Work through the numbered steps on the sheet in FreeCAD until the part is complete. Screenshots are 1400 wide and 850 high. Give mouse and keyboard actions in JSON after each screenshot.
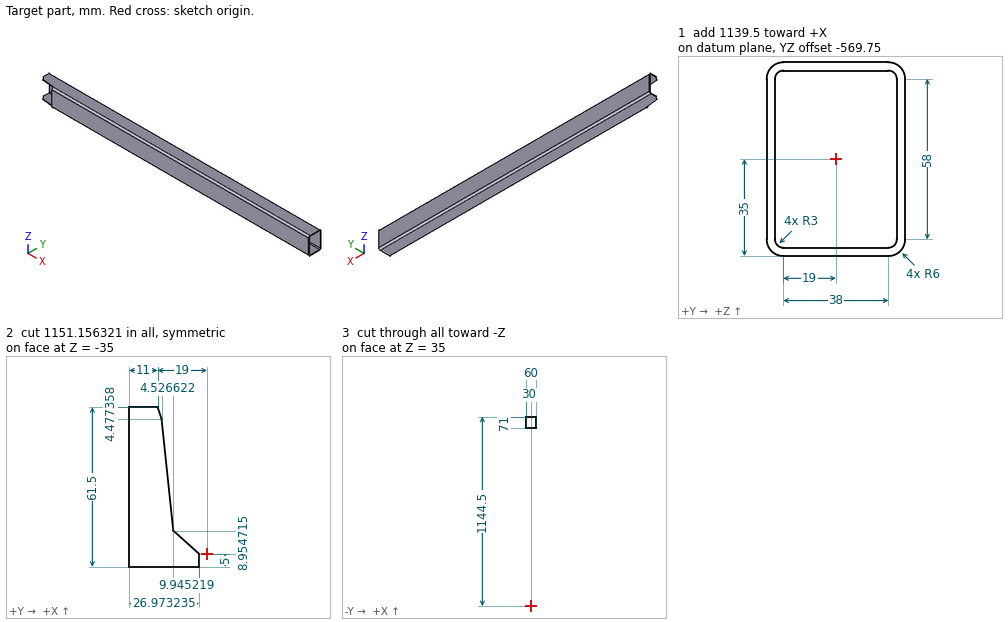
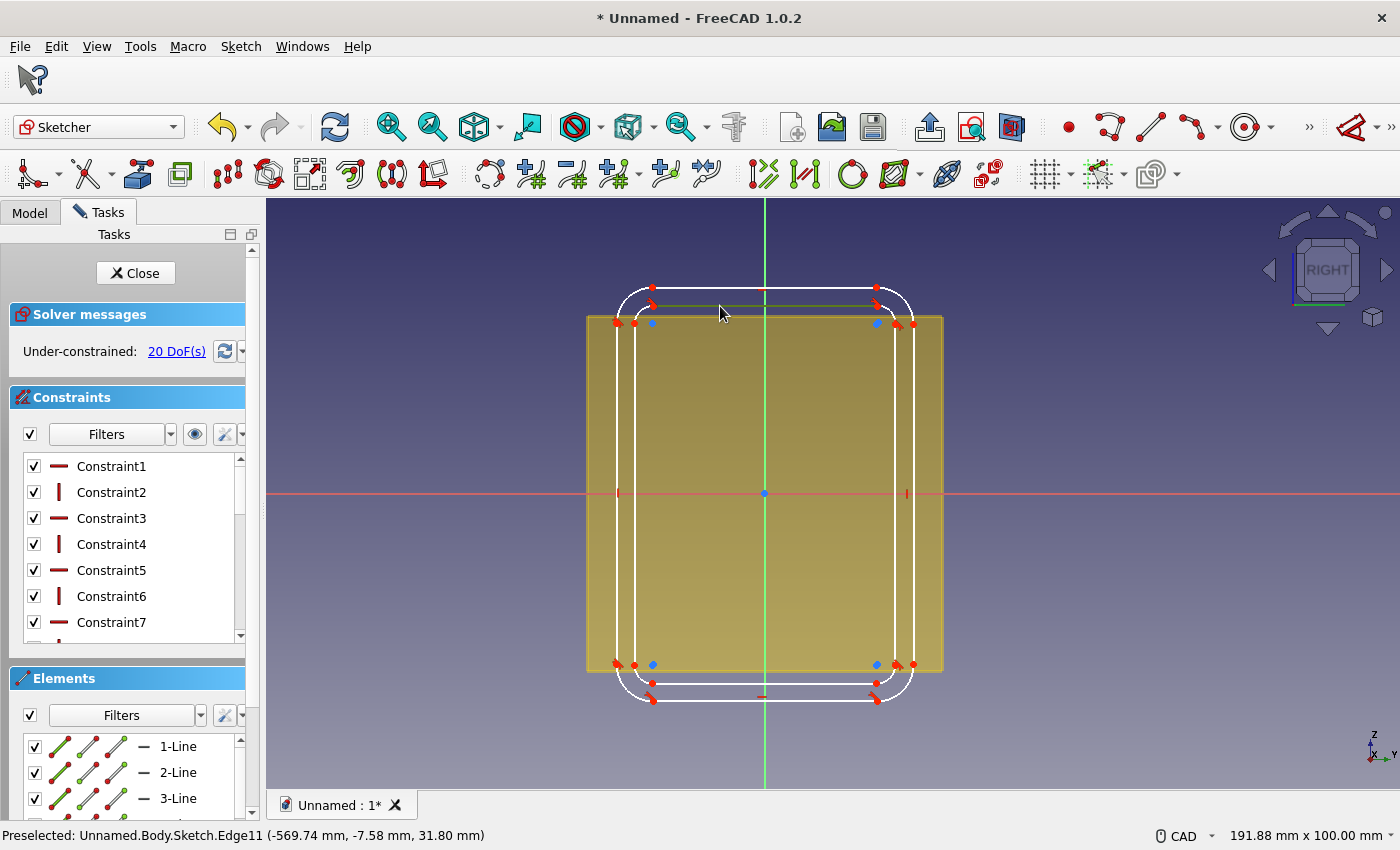
{"action": "left_click", "coordinate": [640, 311]}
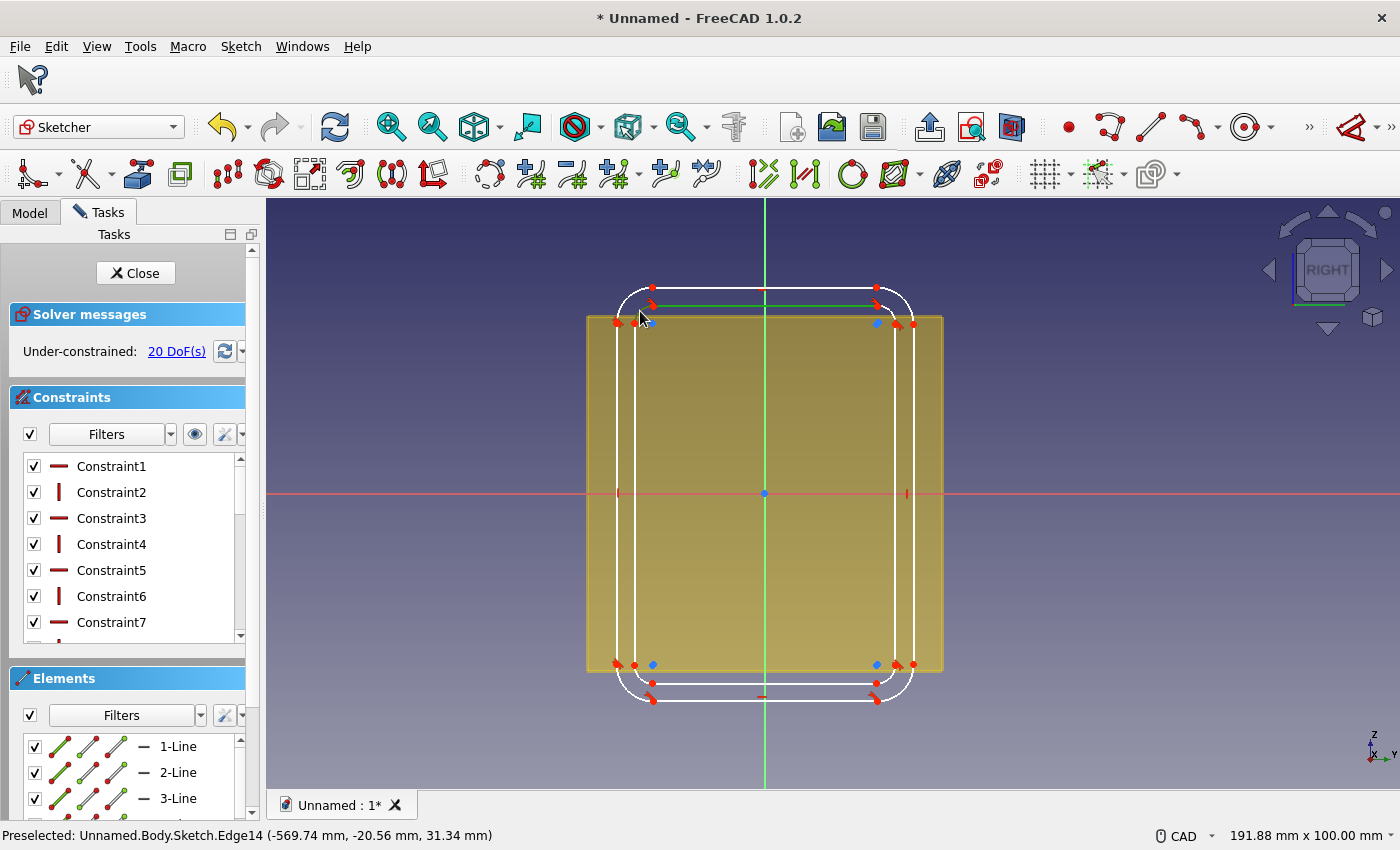
{"action": "key", "text": "t"}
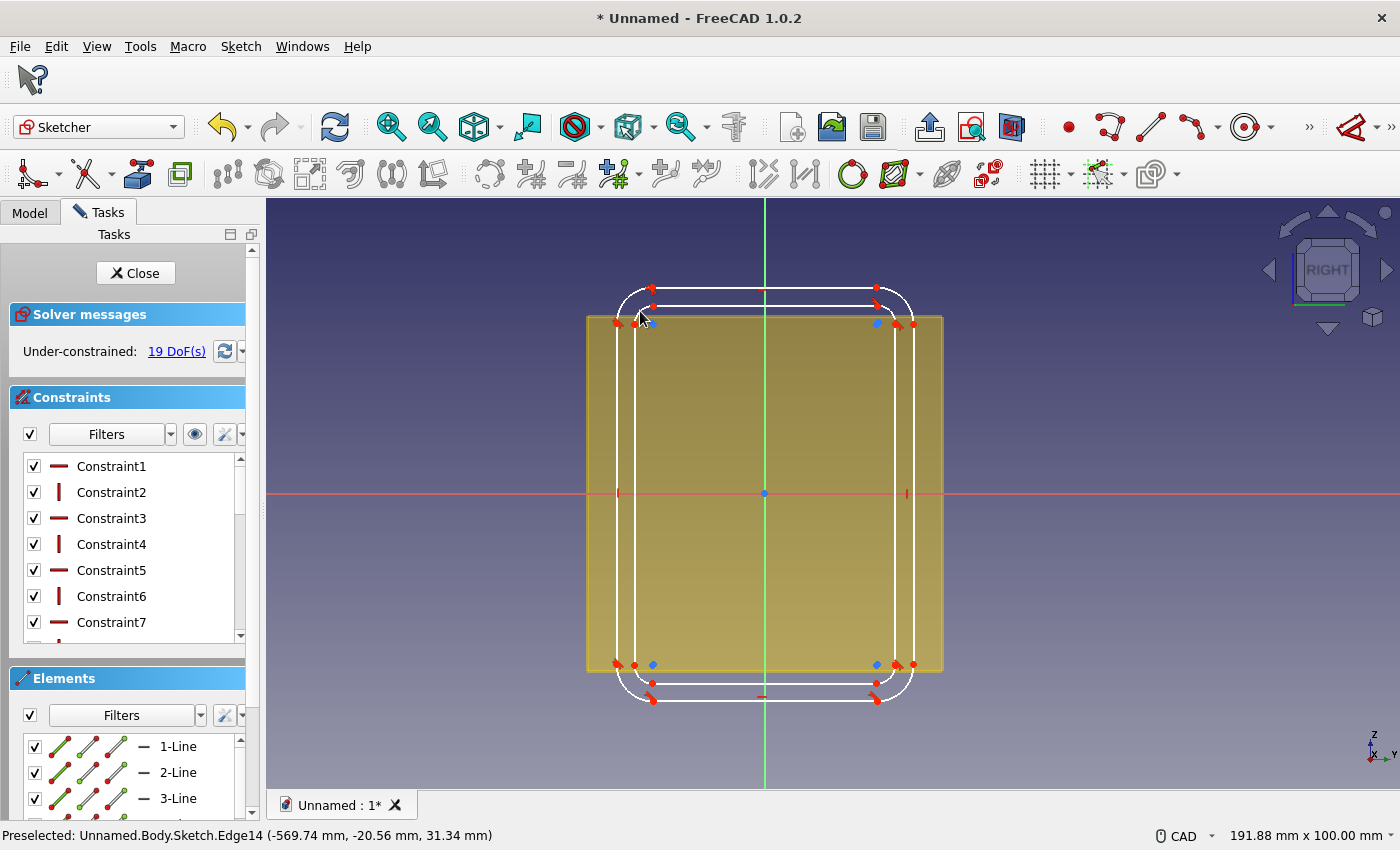
{"action": "left_click", "coordinate": [720, 306]}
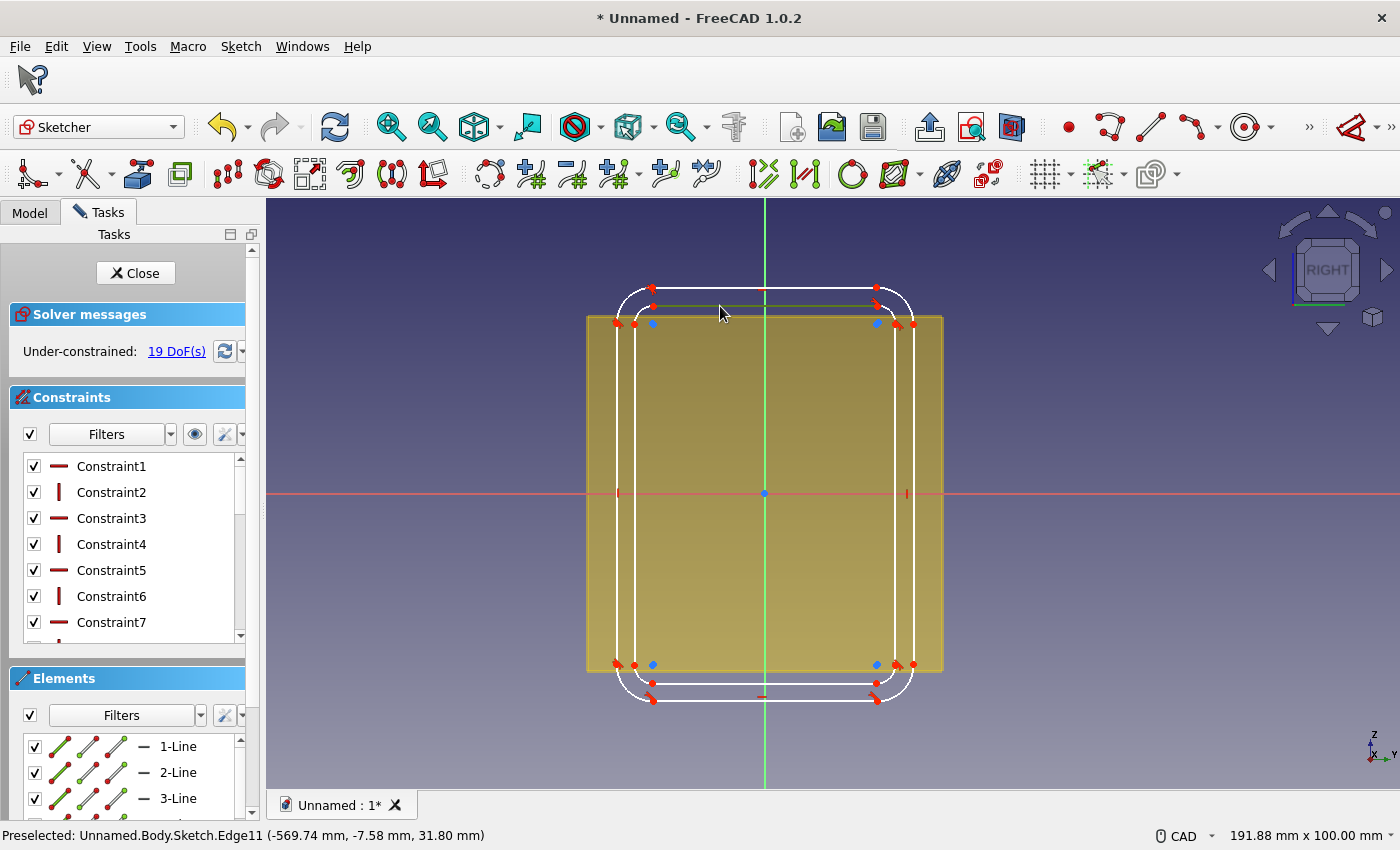
{"action": "left_click", "coordinate": [890, 311]}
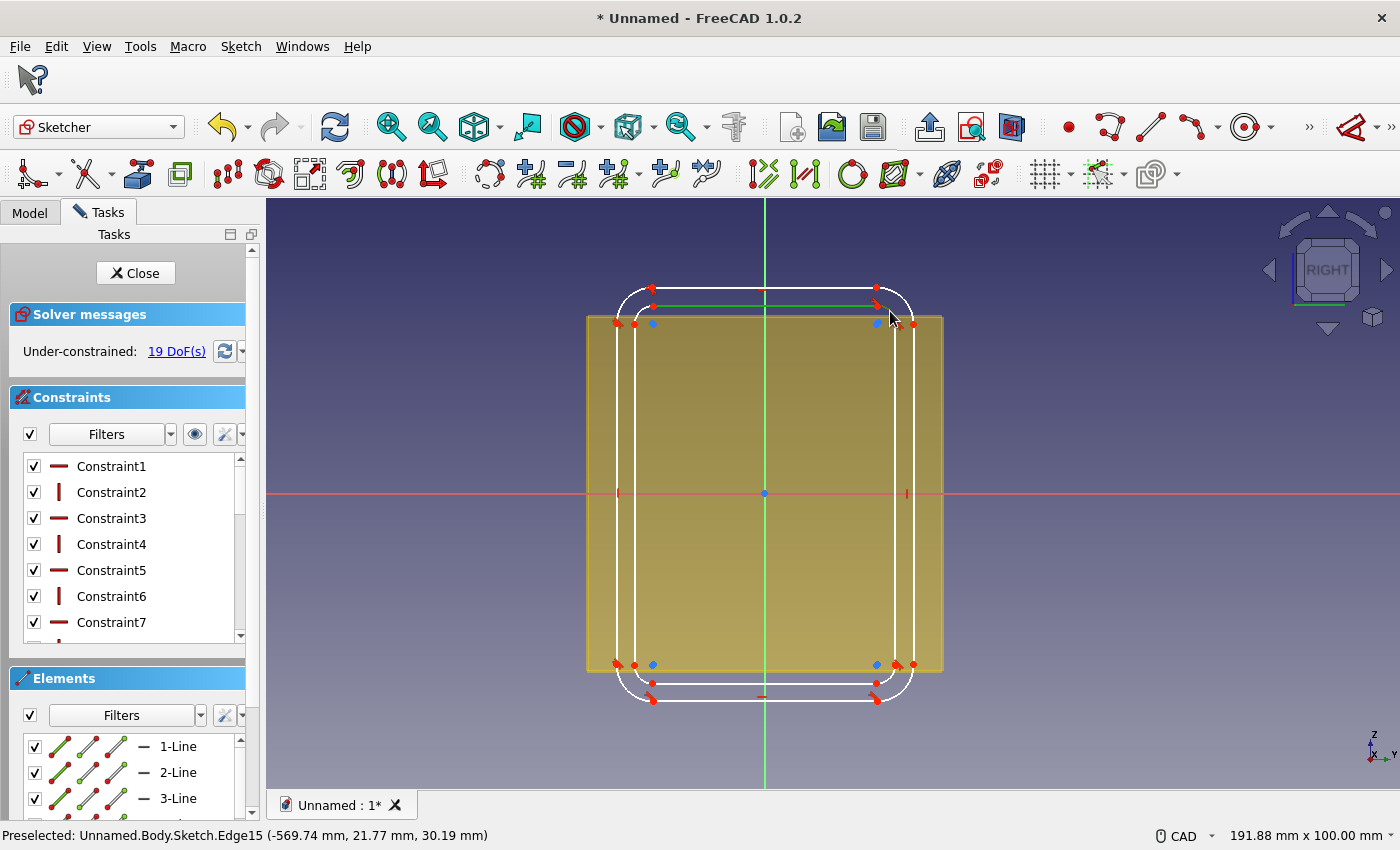
{"action": "key", "text": "t"}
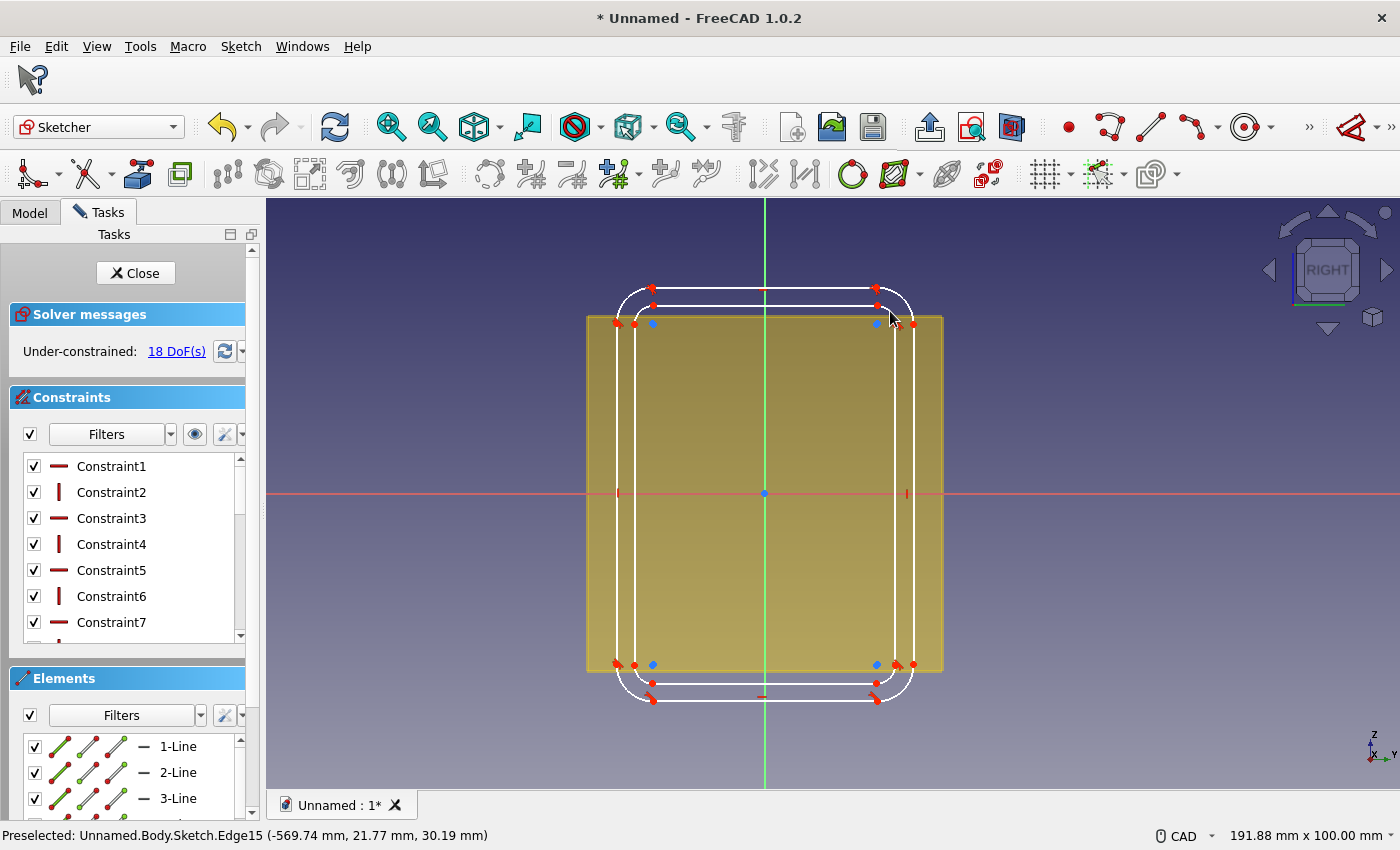
{"action": "left_click", "coordinate": [895, 427]}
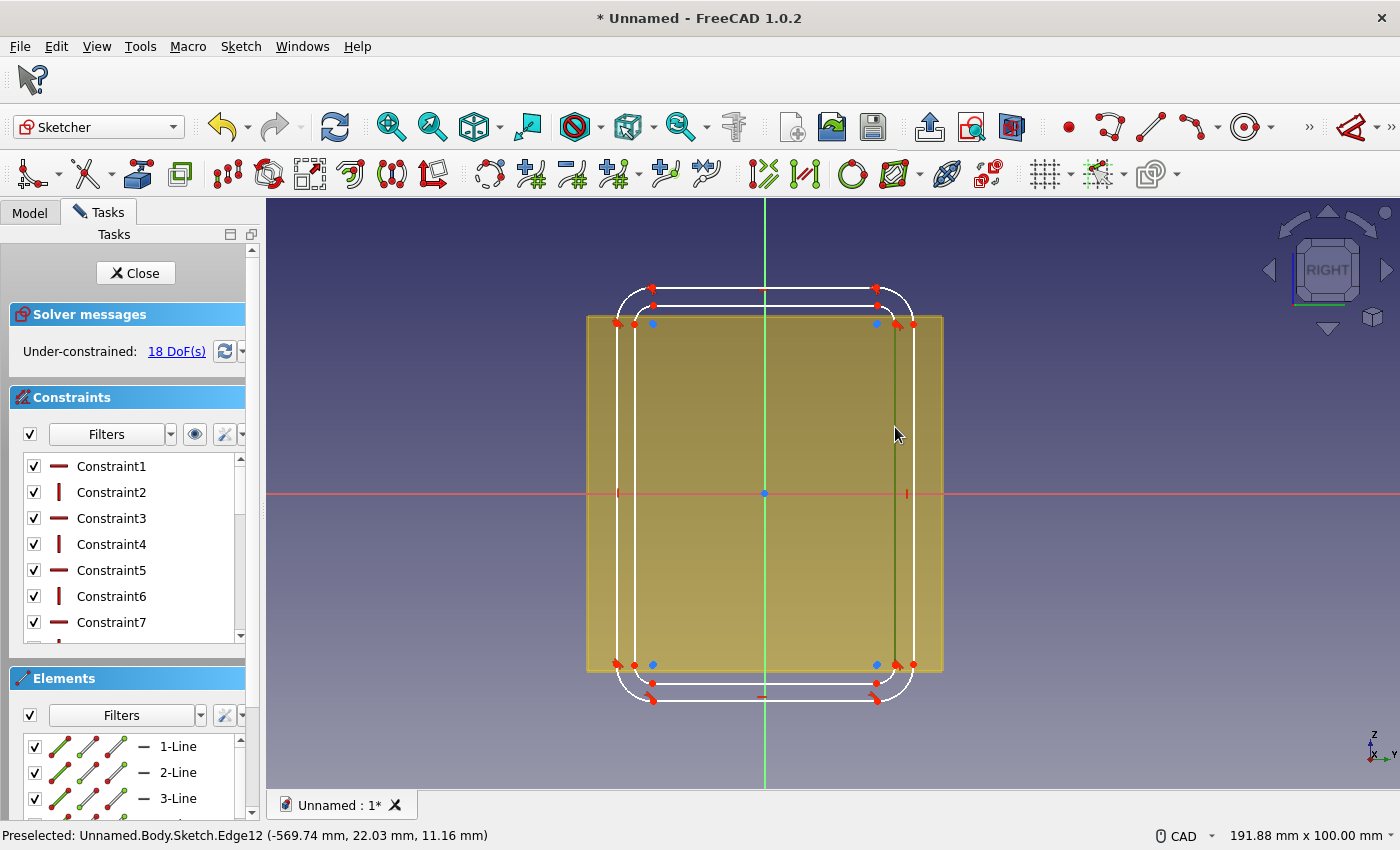
{"action": "left_click", "coordinate": [890, 311]}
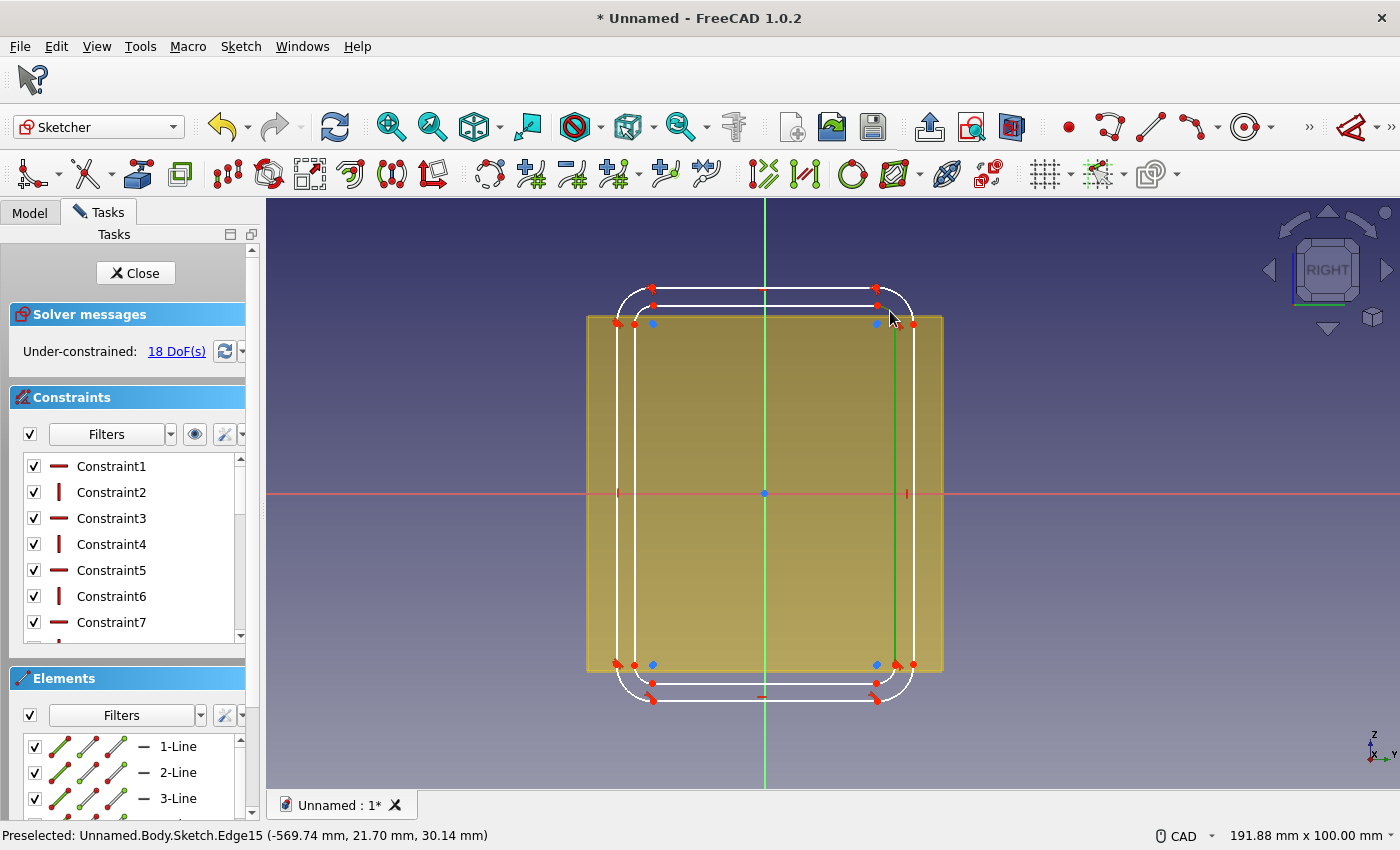
{"action": "key", "text": "t"}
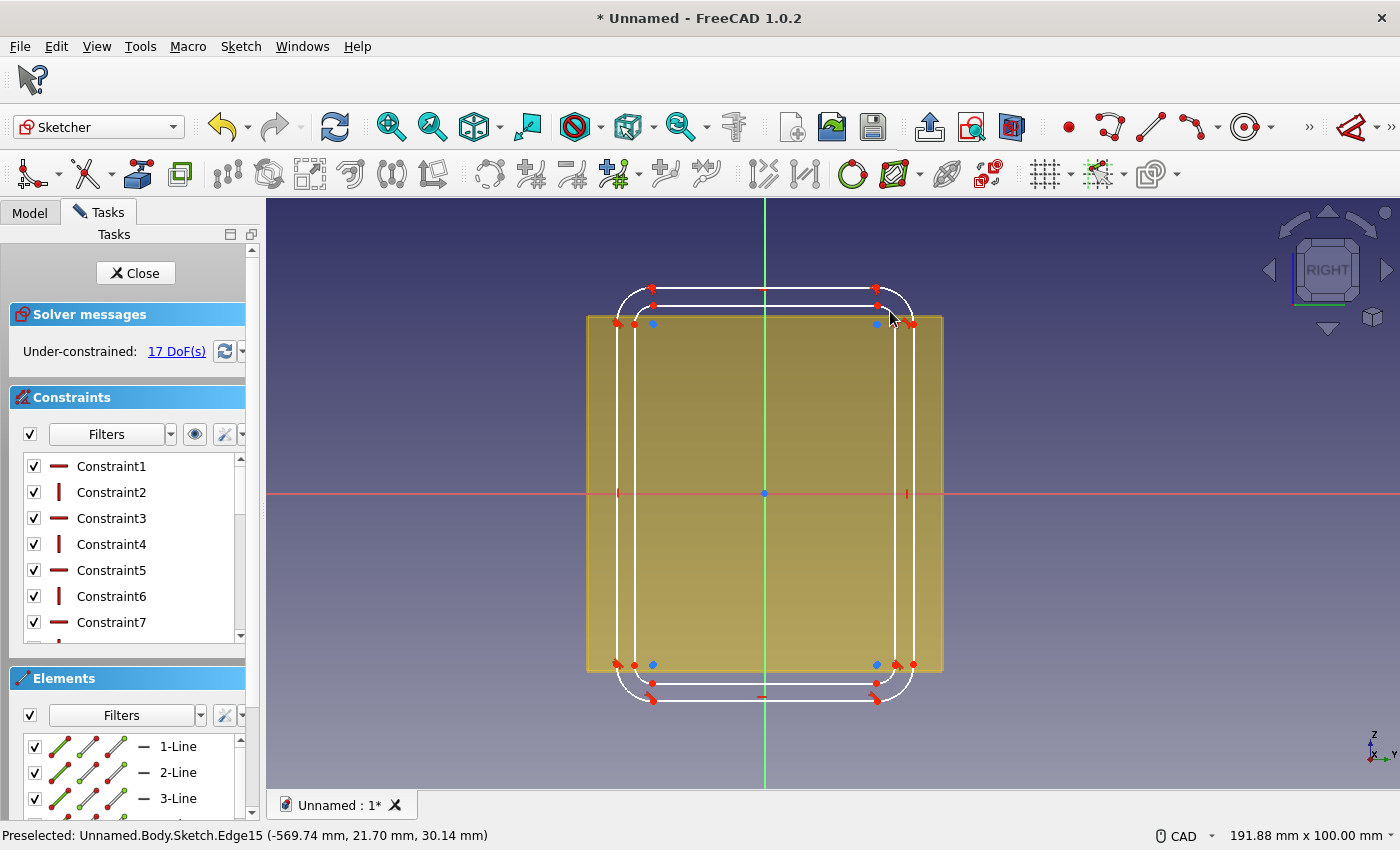
{"action": "left_click", "coordinate": [895, 427]}